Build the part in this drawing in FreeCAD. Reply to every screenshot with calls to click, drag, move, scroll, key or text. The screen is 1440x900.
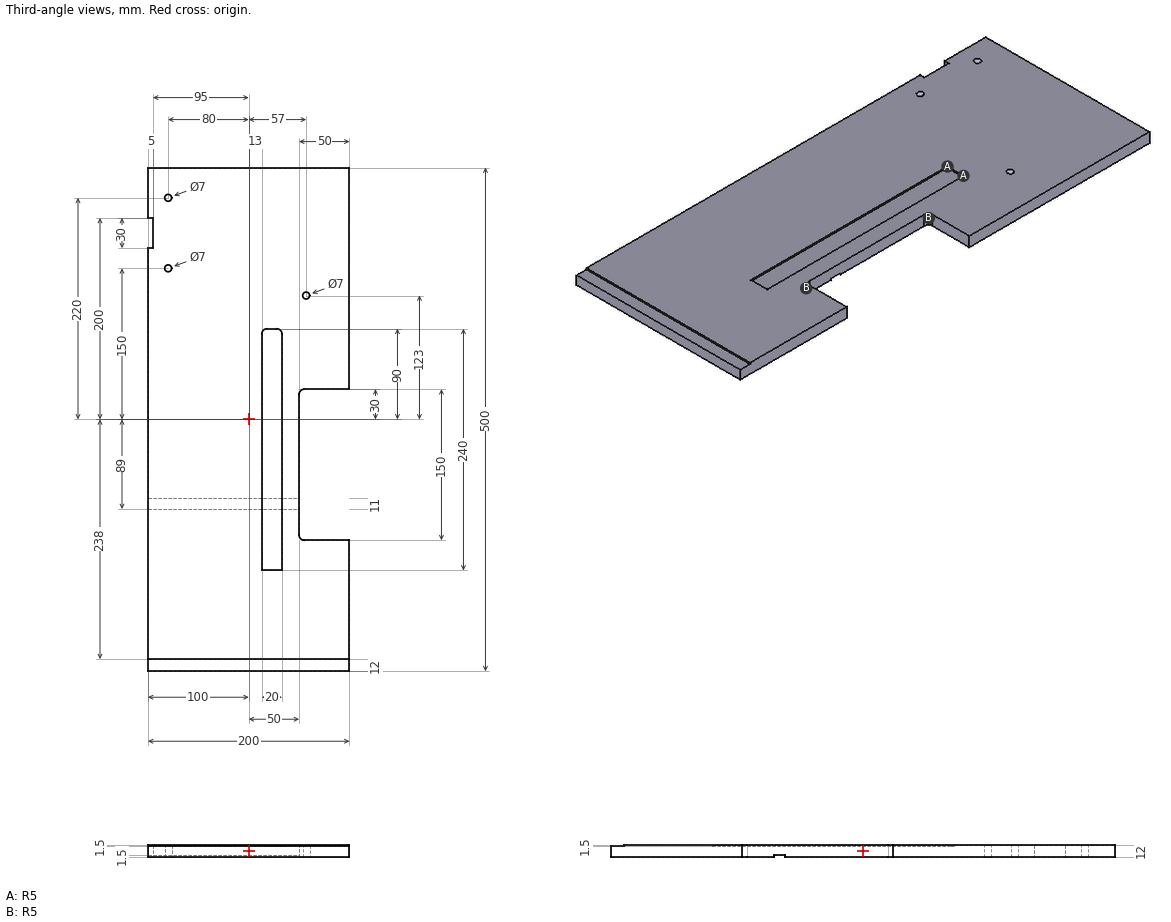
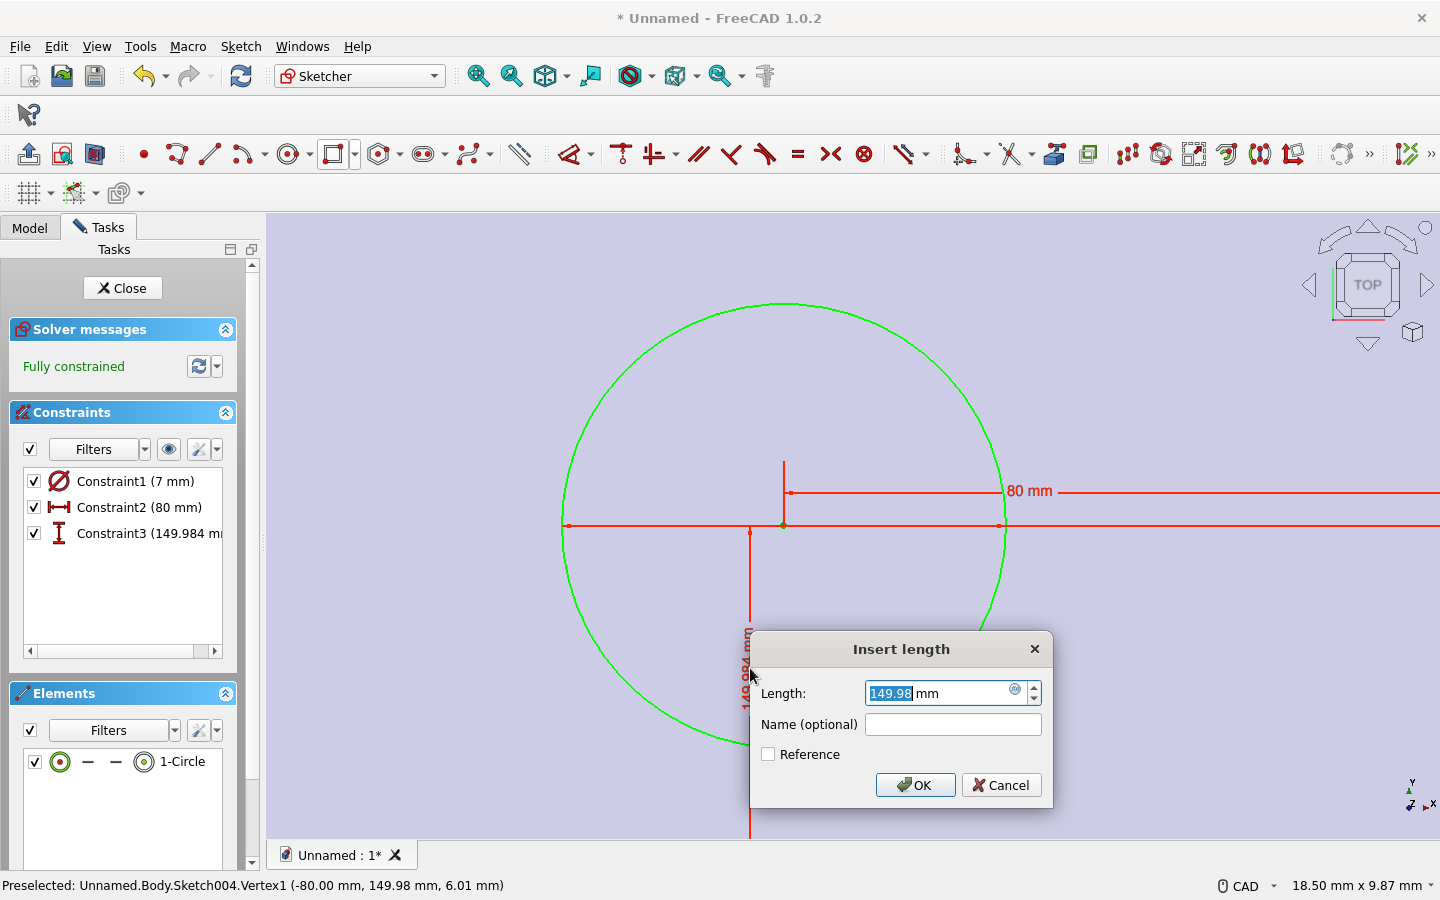
text(150)
key(Return)
key(Escape)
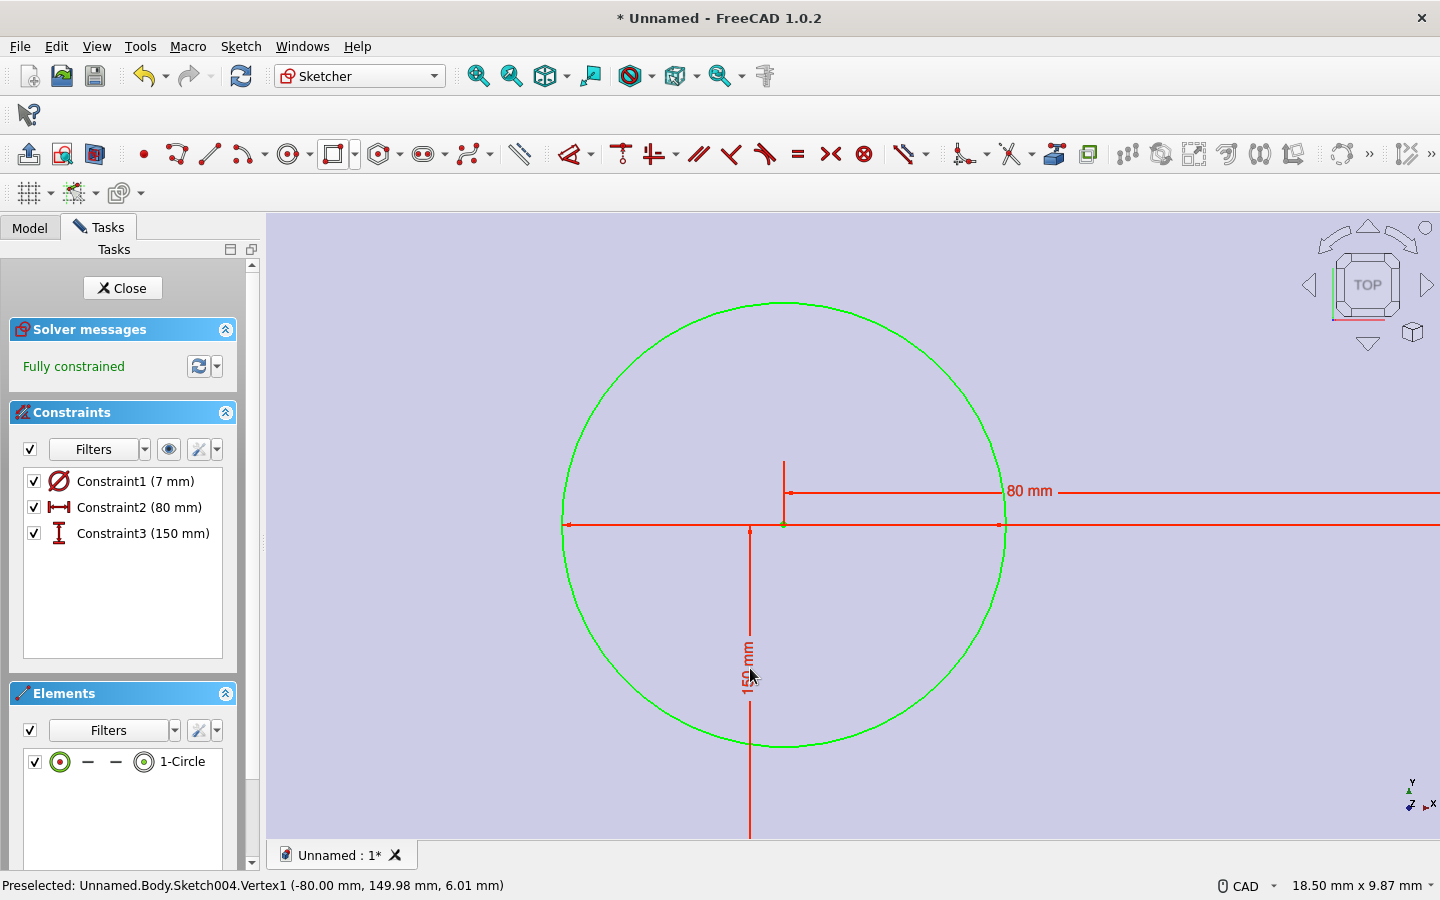
click(123, 288)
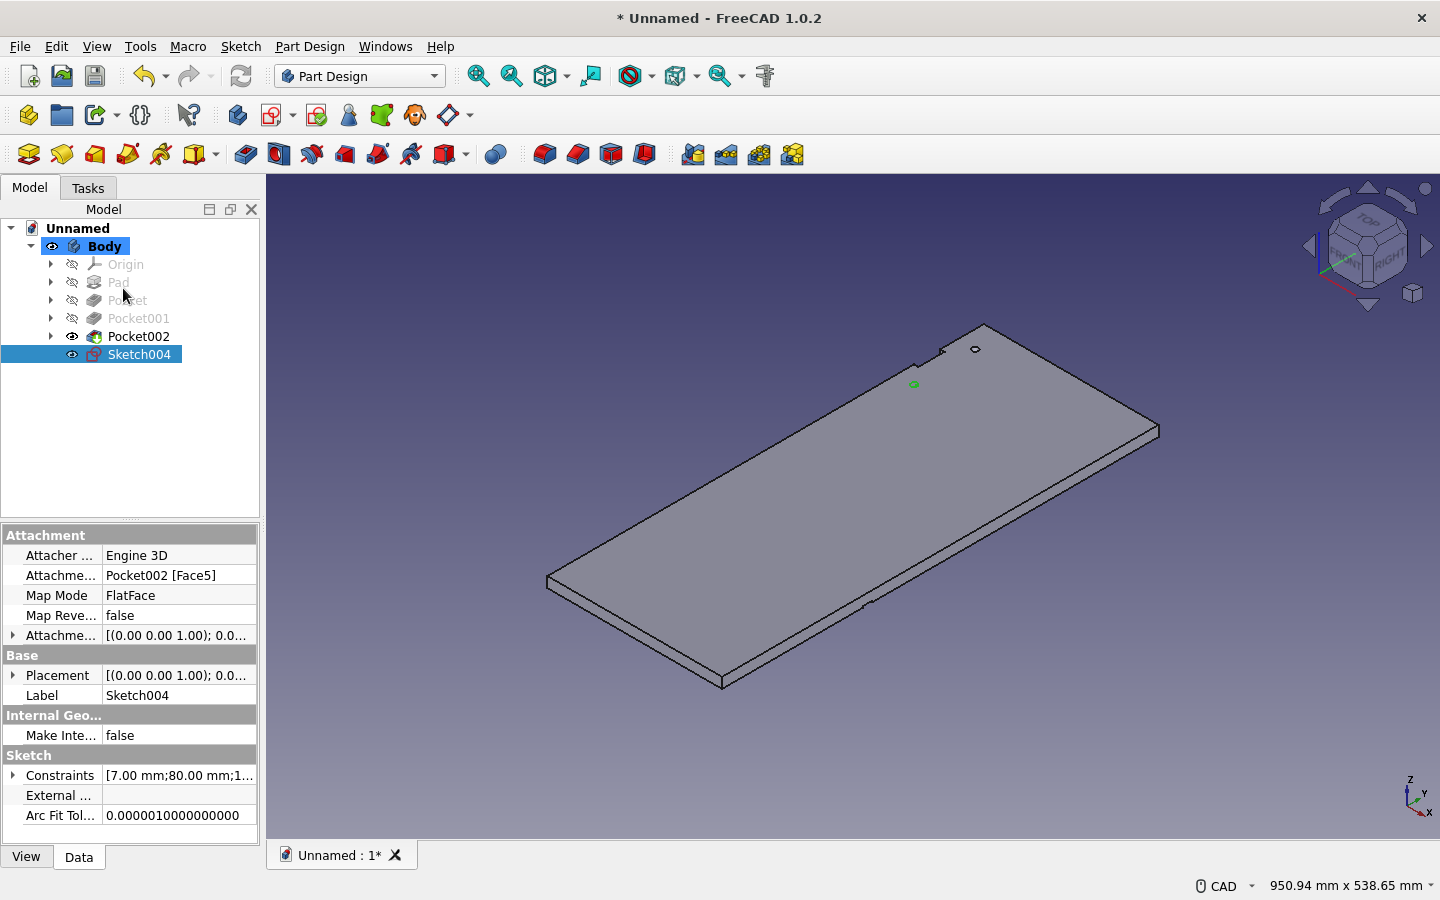
click(246, 154)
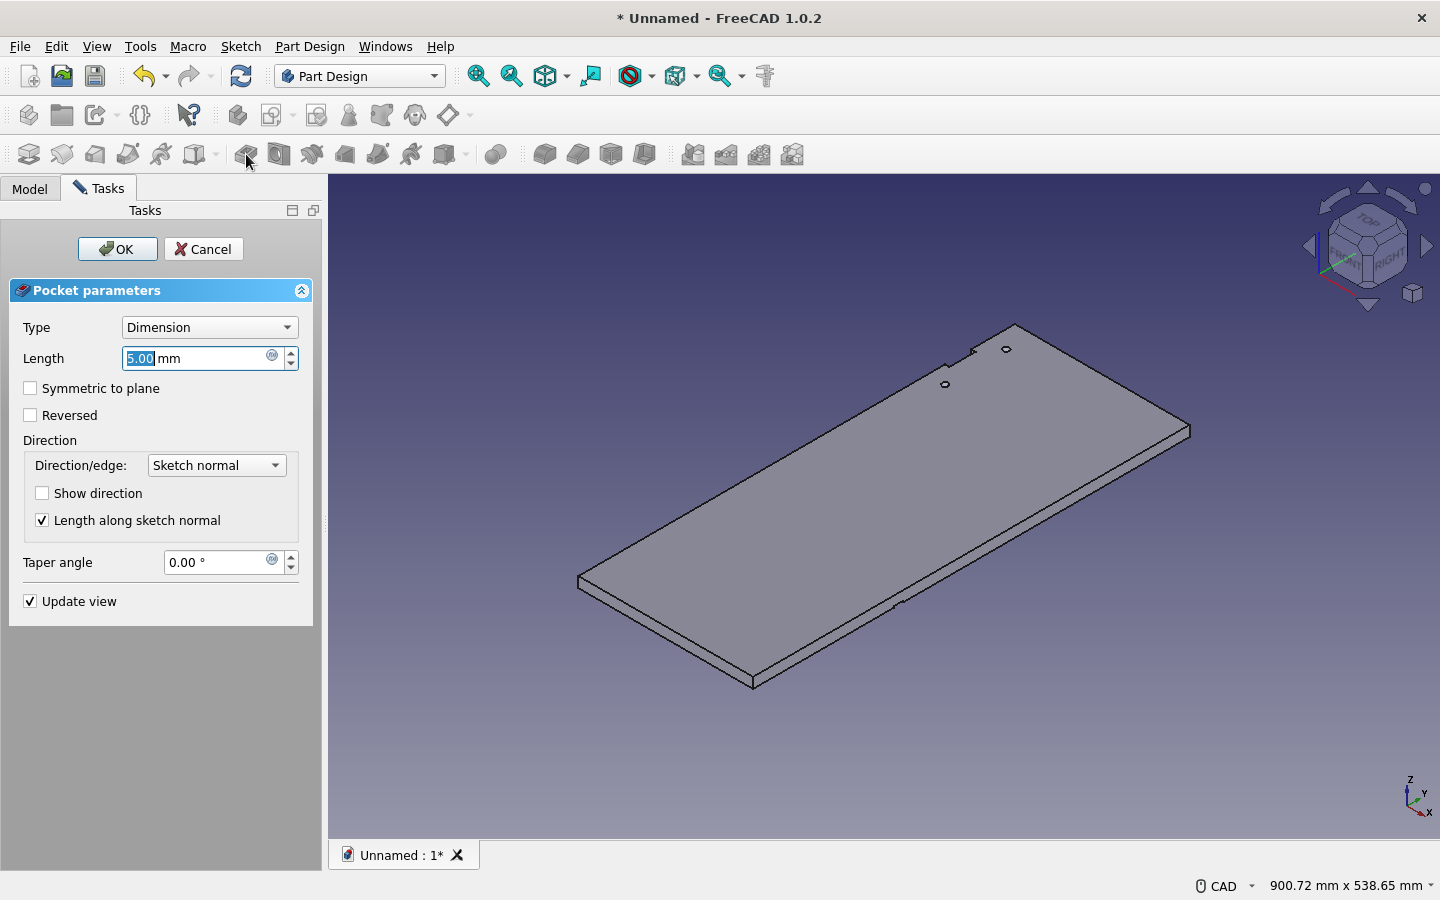
click(210, 328)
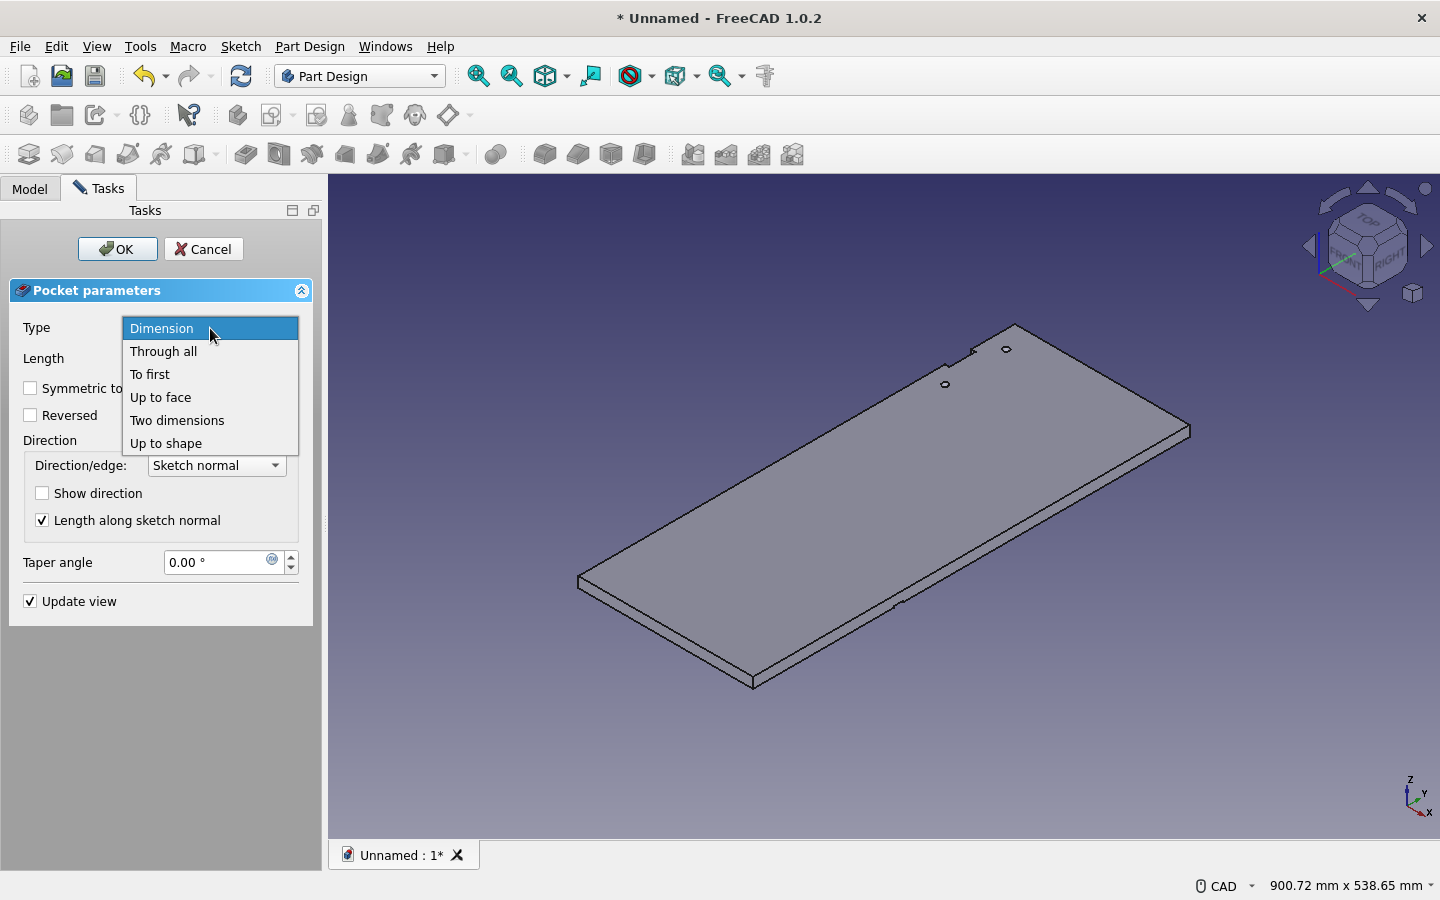
click(208, 374)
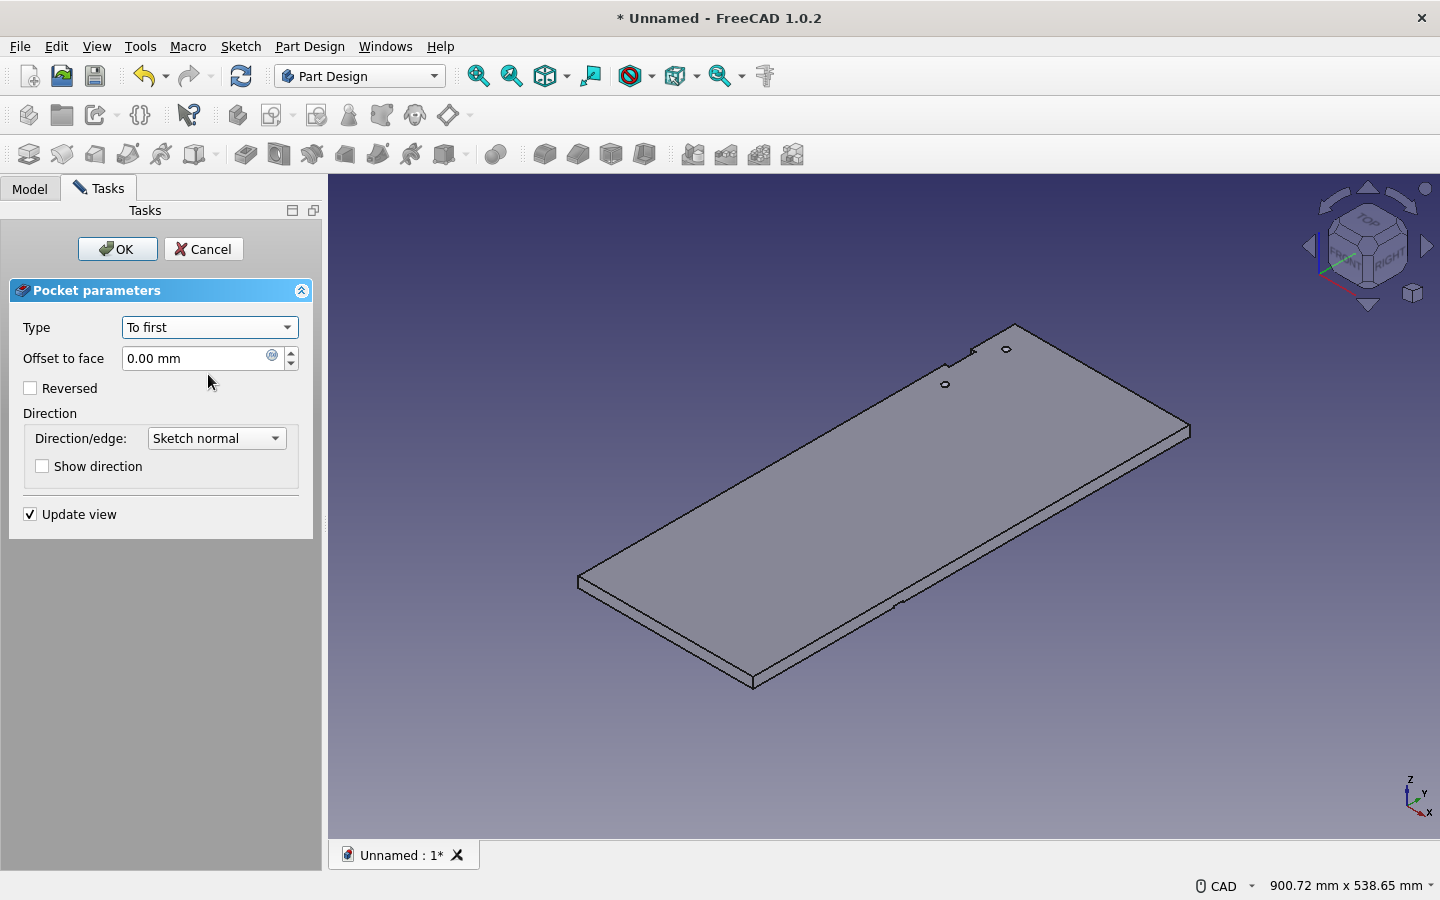
click(118, 249)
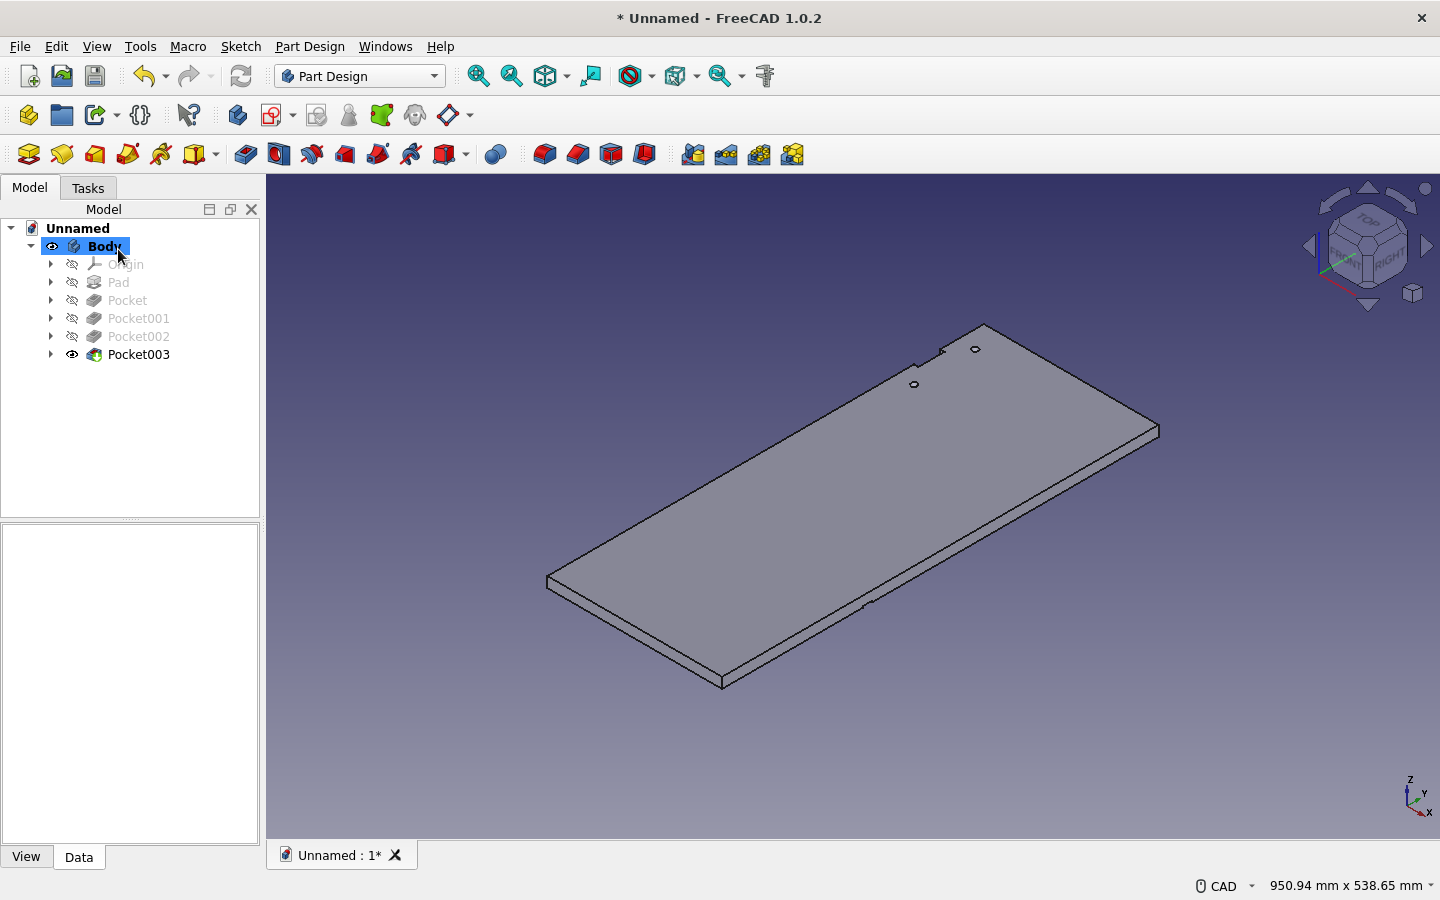
click(915, 463)